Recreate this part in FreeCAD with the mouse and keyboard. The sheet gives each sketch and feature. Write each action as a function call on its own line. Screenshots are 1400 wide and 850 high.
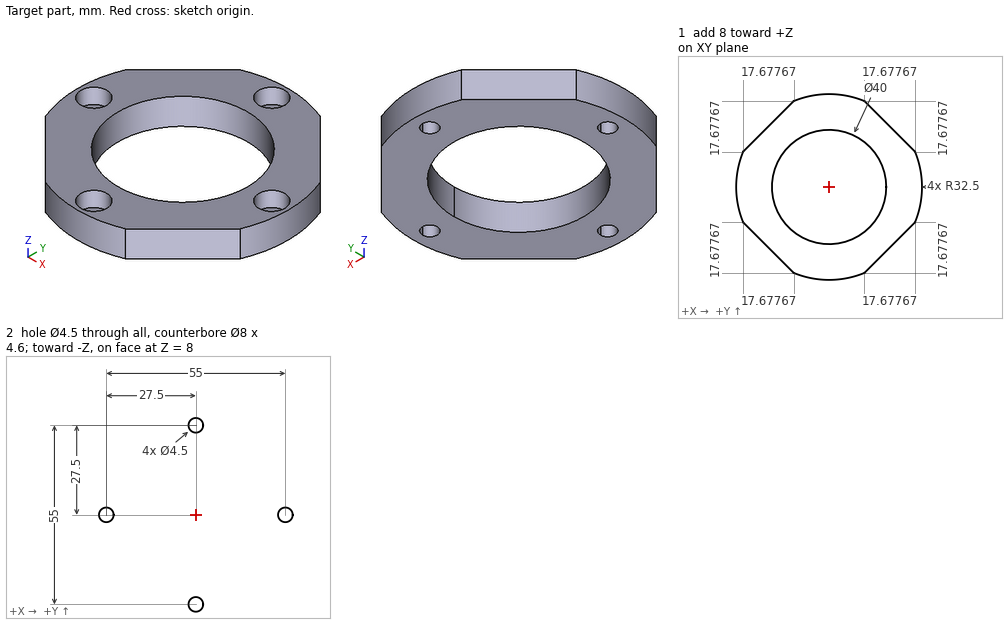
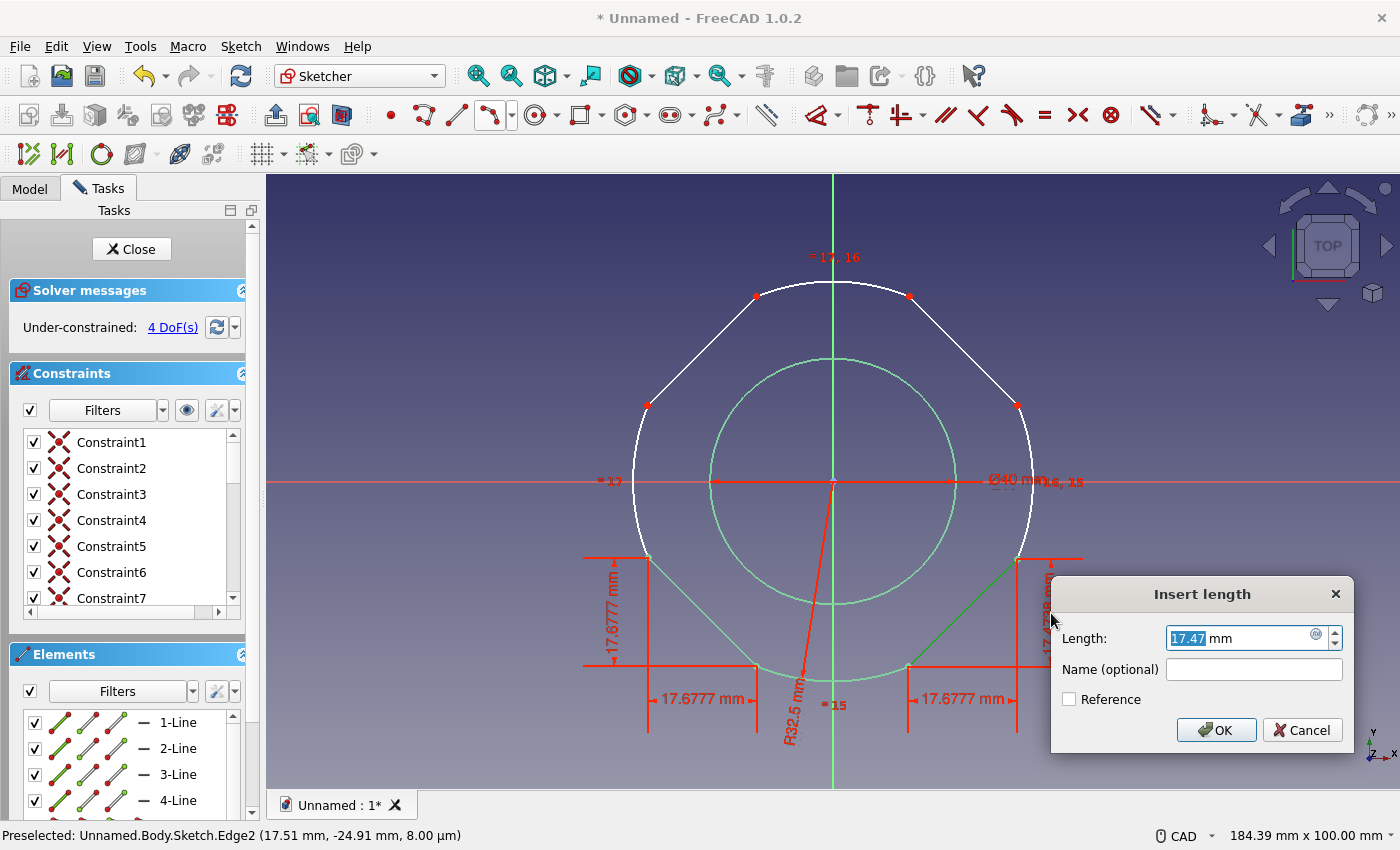
text(17.67767)
key(Return)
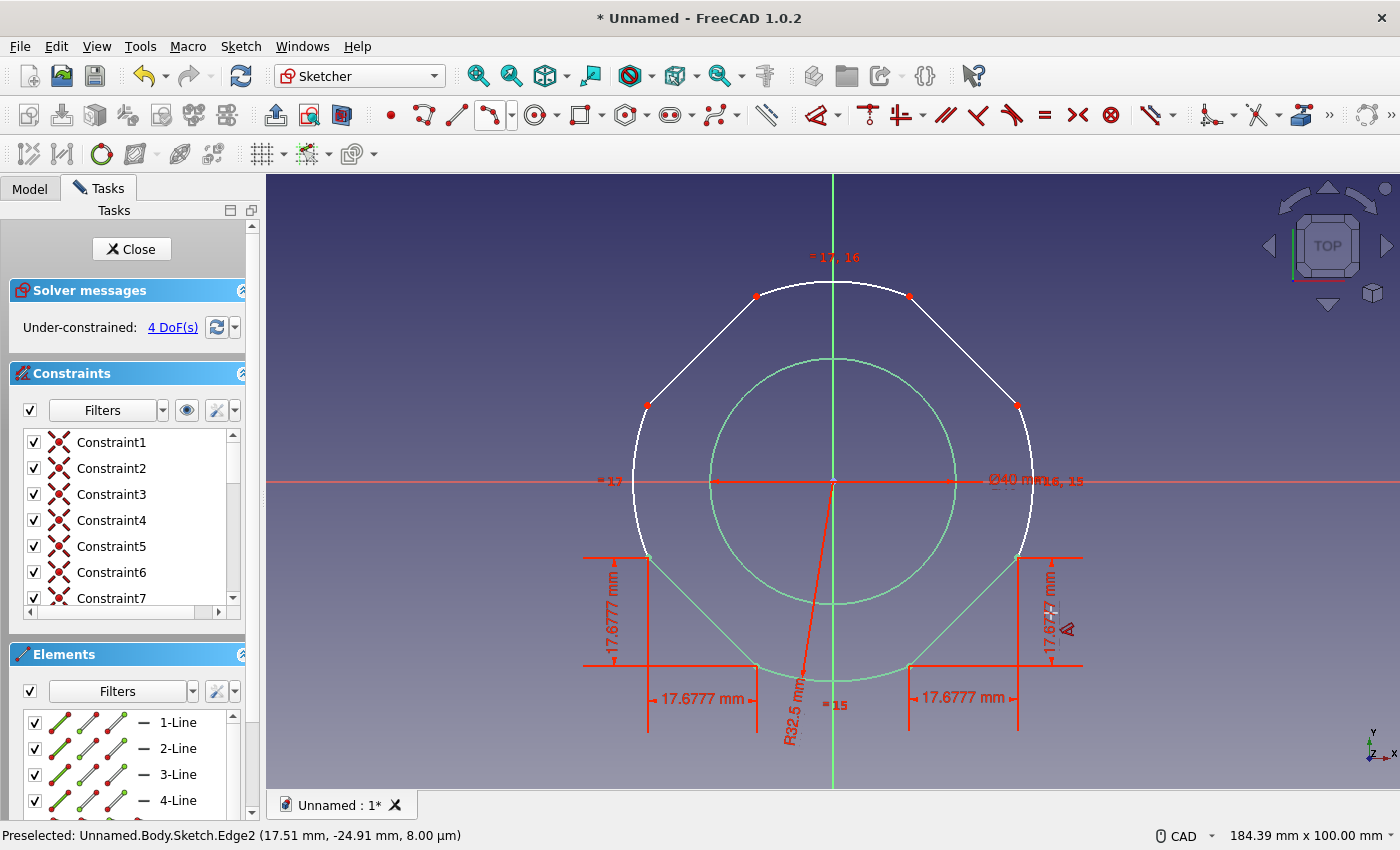
click(985, 373)
click(964, 263)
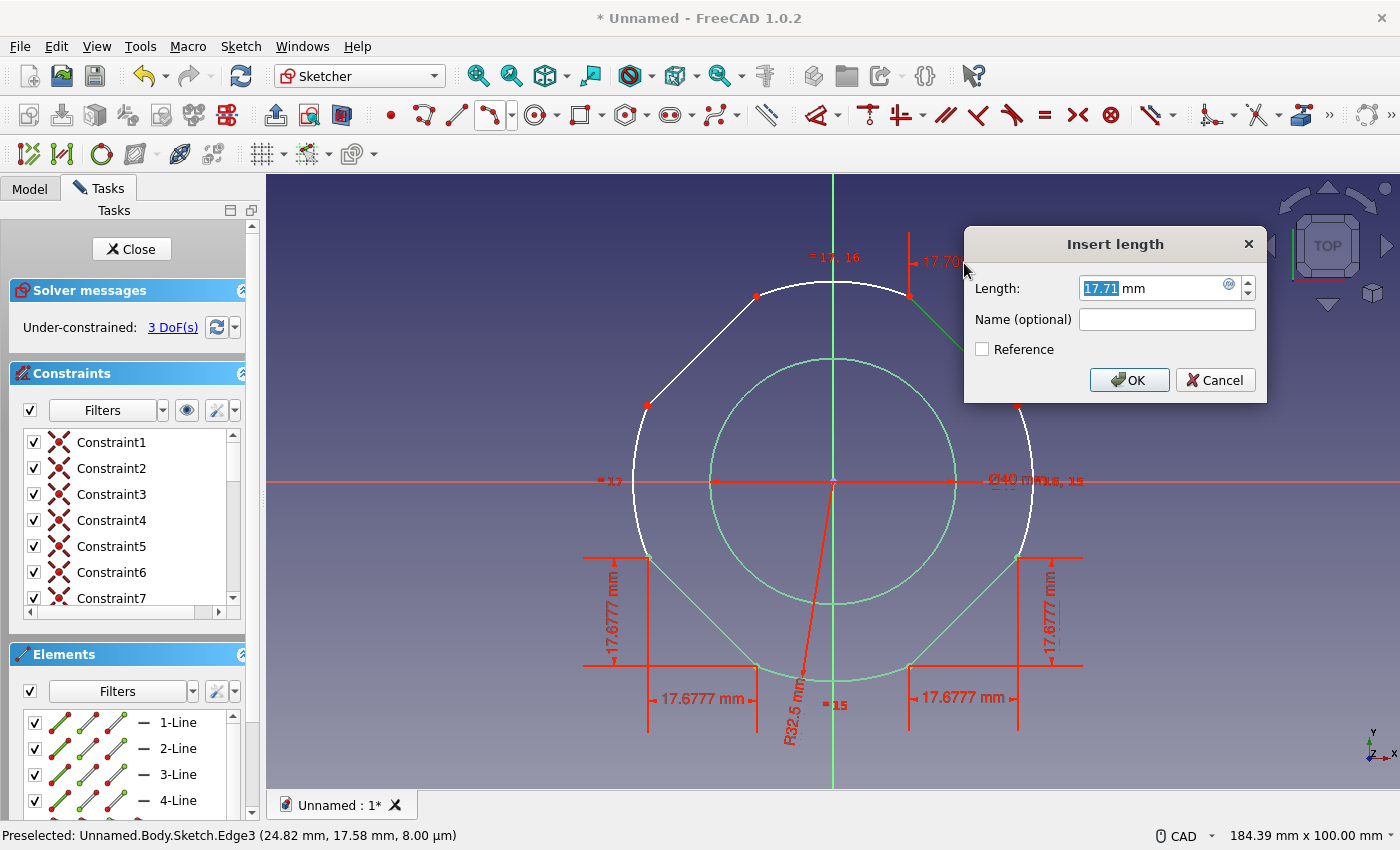
text(17.67767)
key(Return)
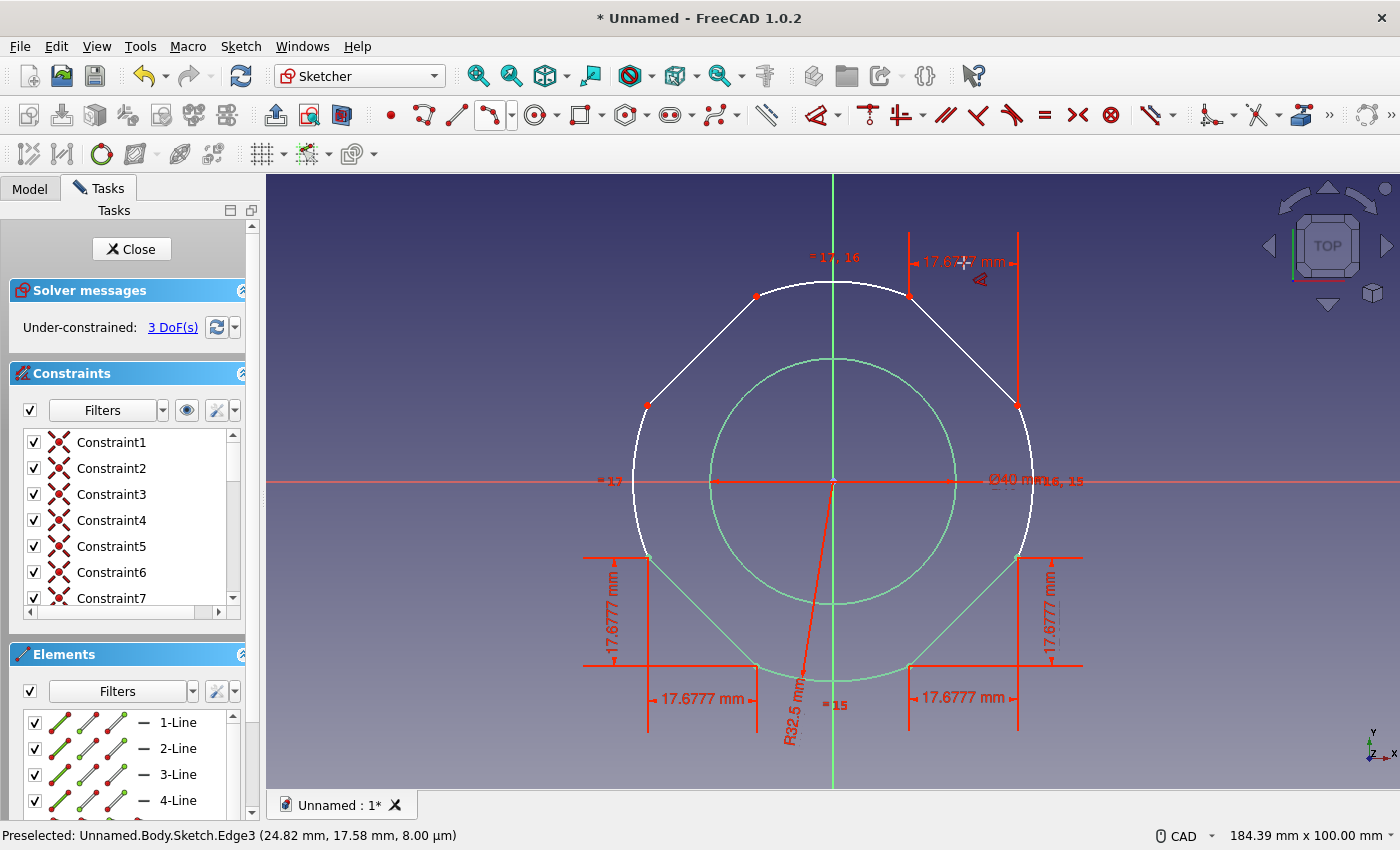
click(985, 373)
click(1052, 351)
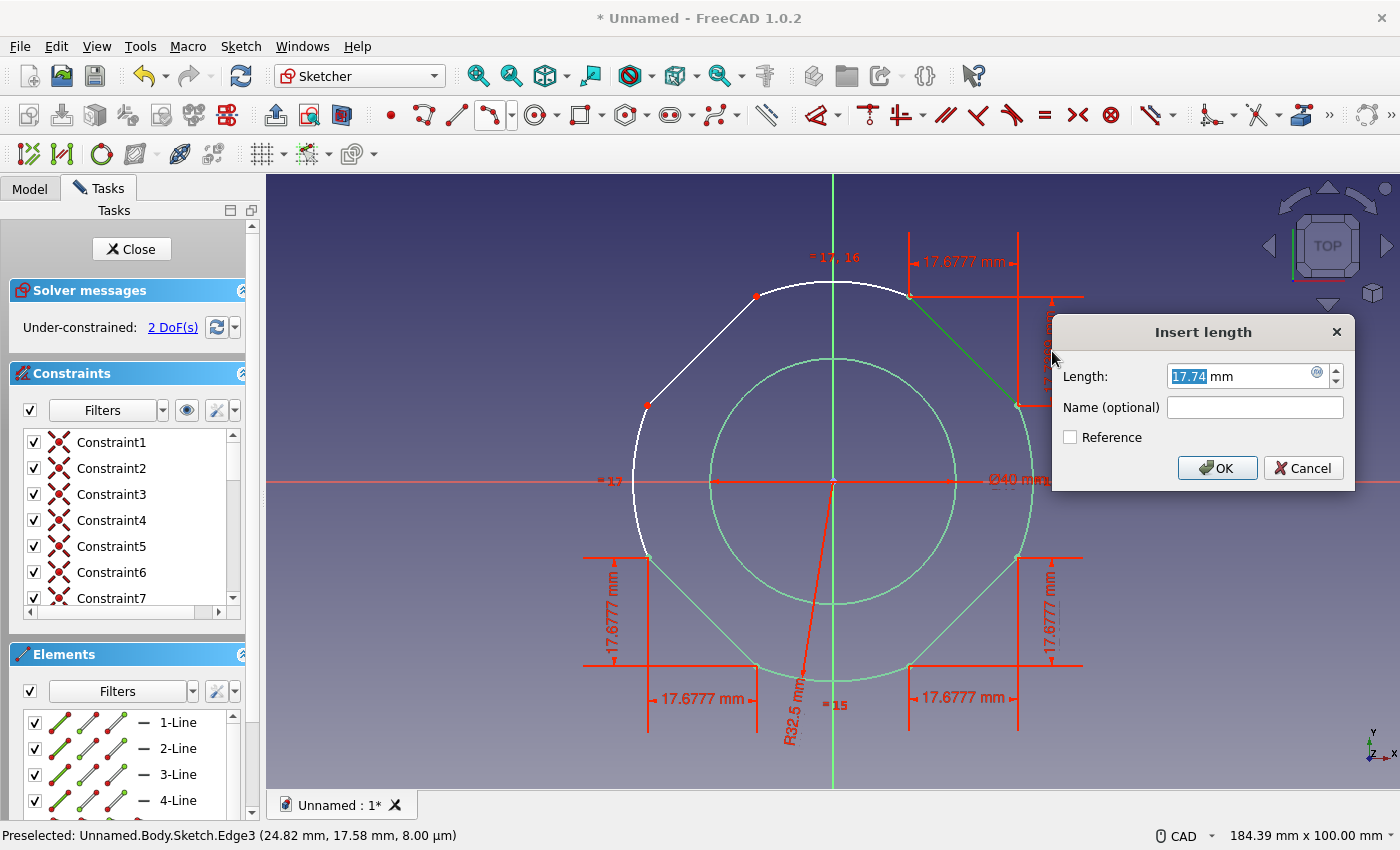
text(17.67767)
key(Return)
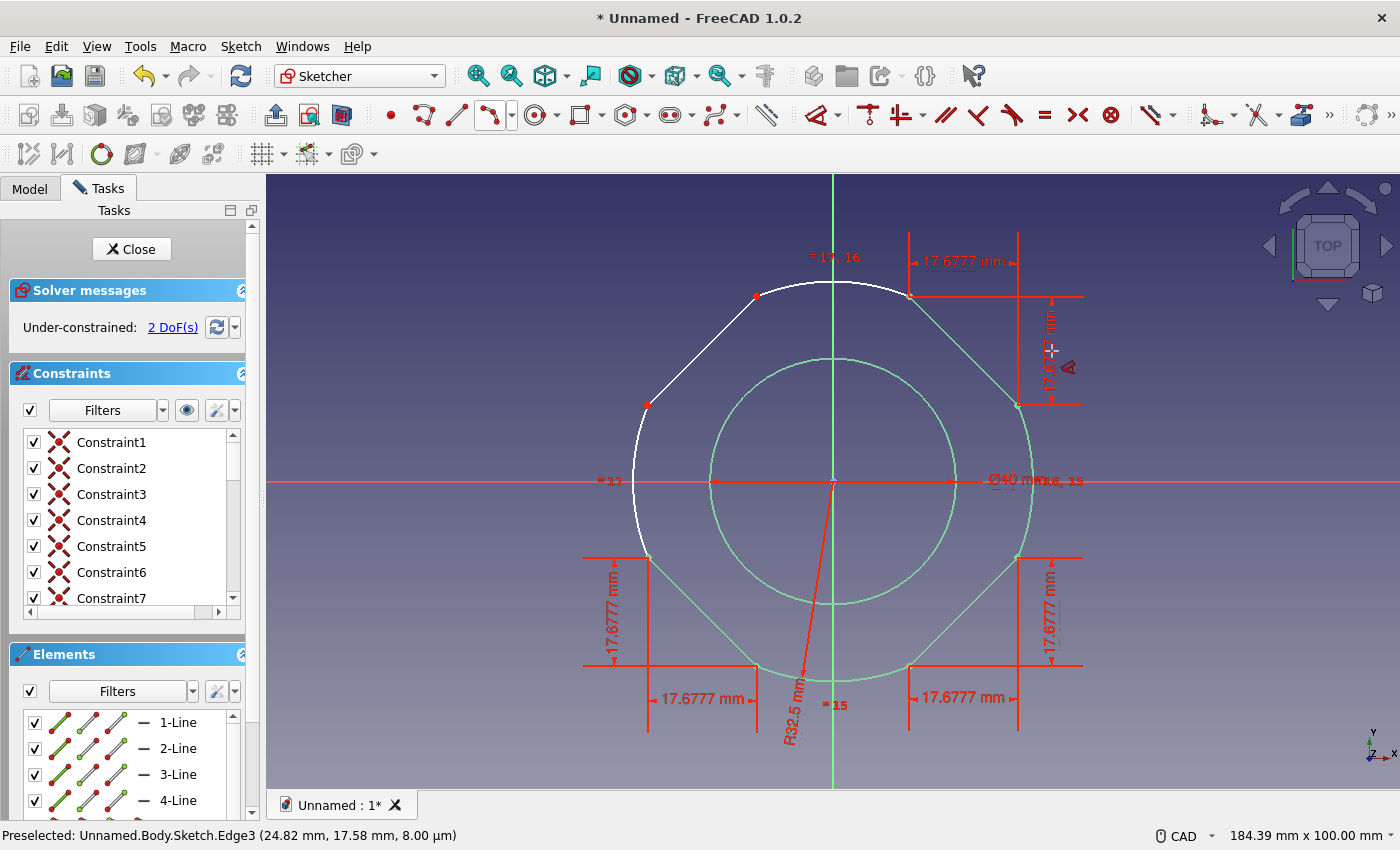
click(724, 329)
click(702, 263)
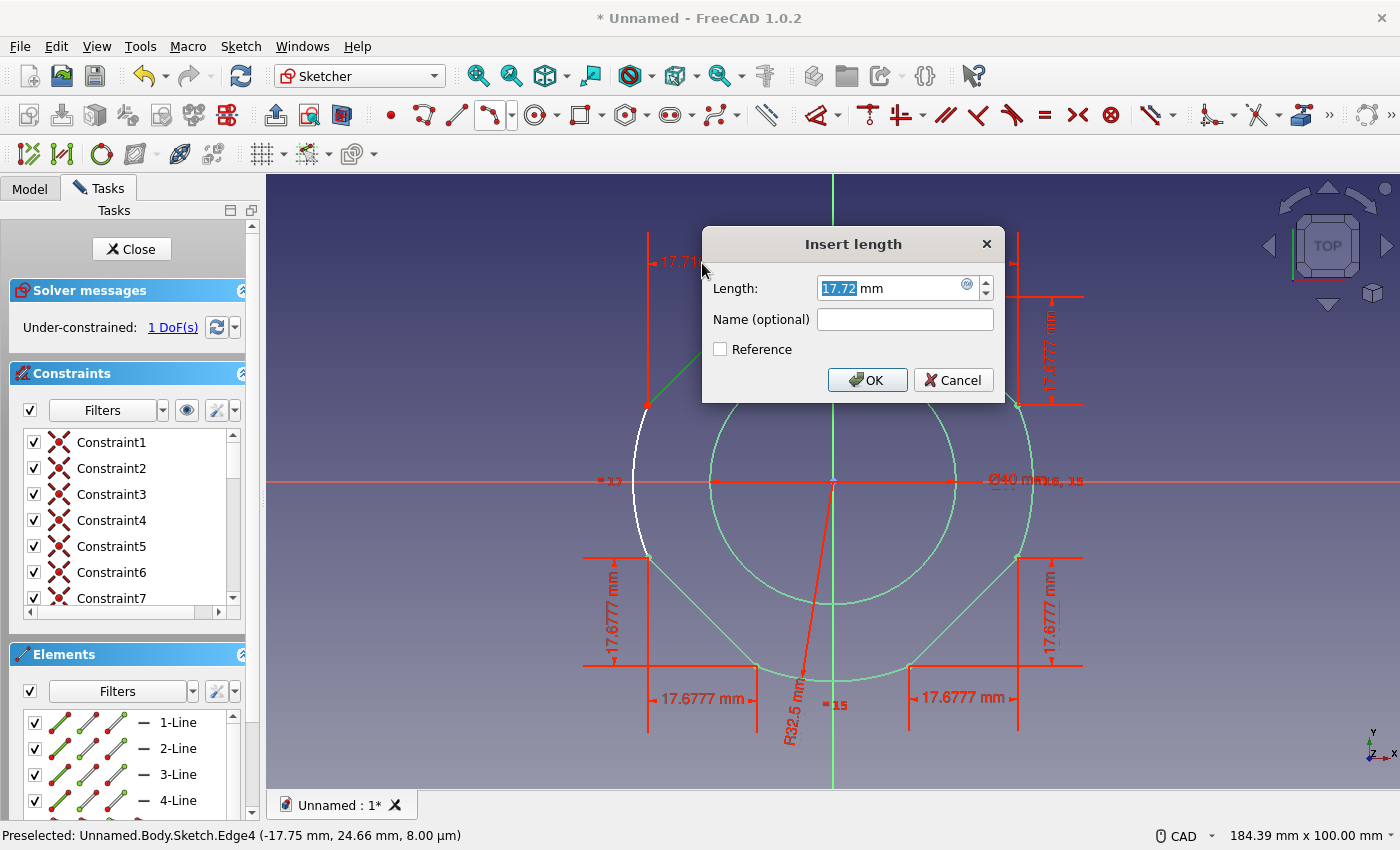
text(17.67767)
key(Return)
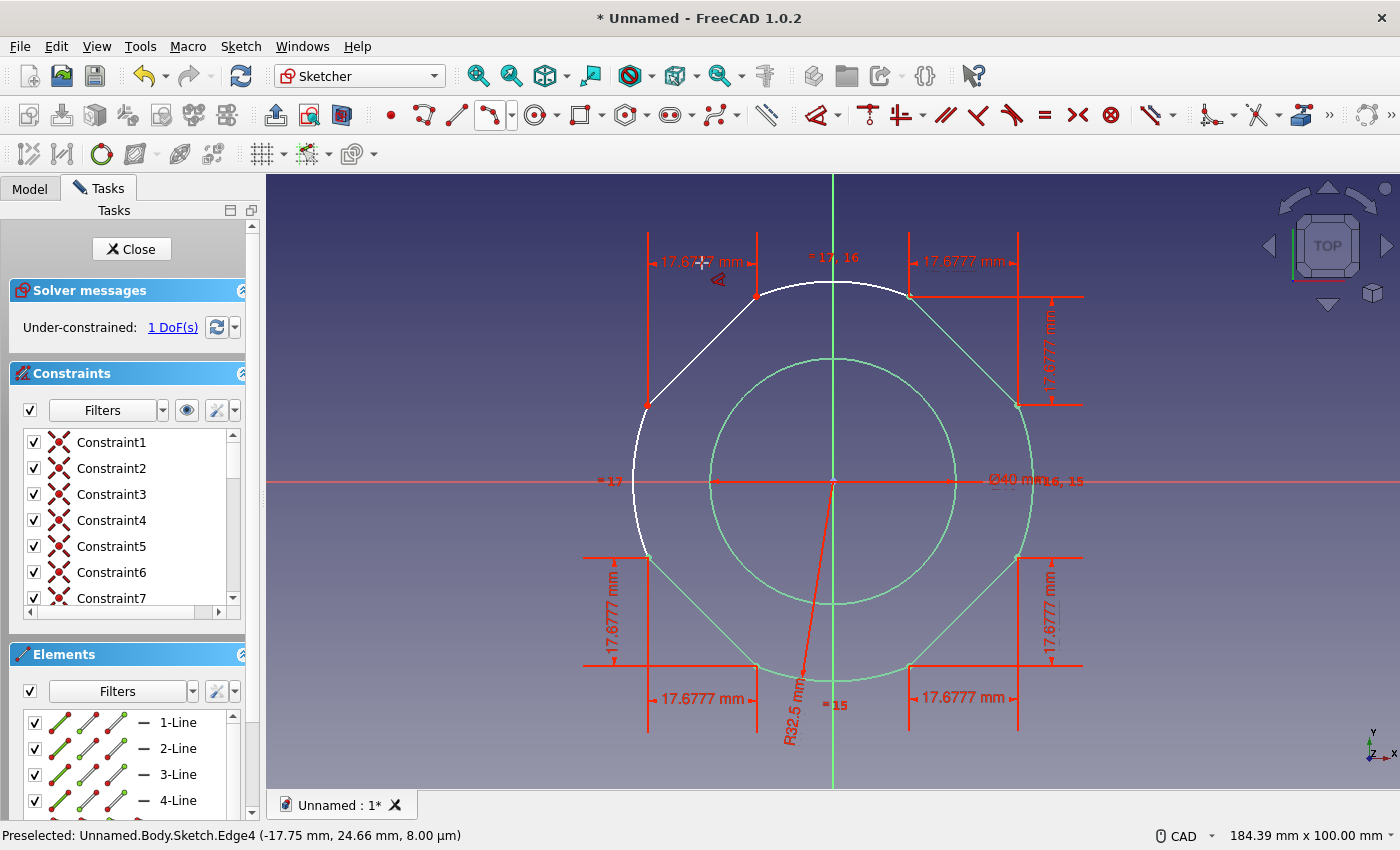
click(724, 330)
click(614, 351)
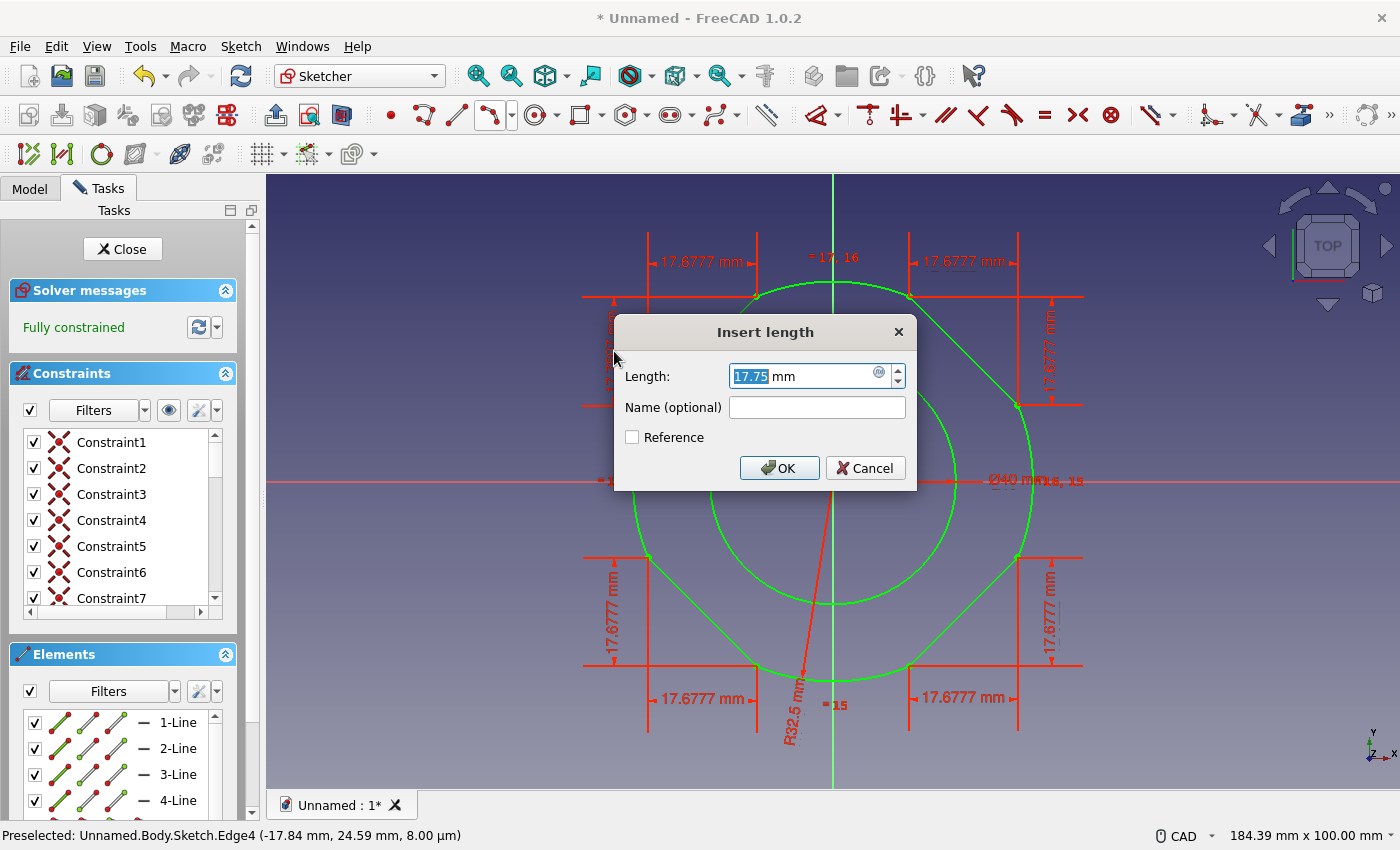
text(17.67767)
key(Return)
key(Escape)